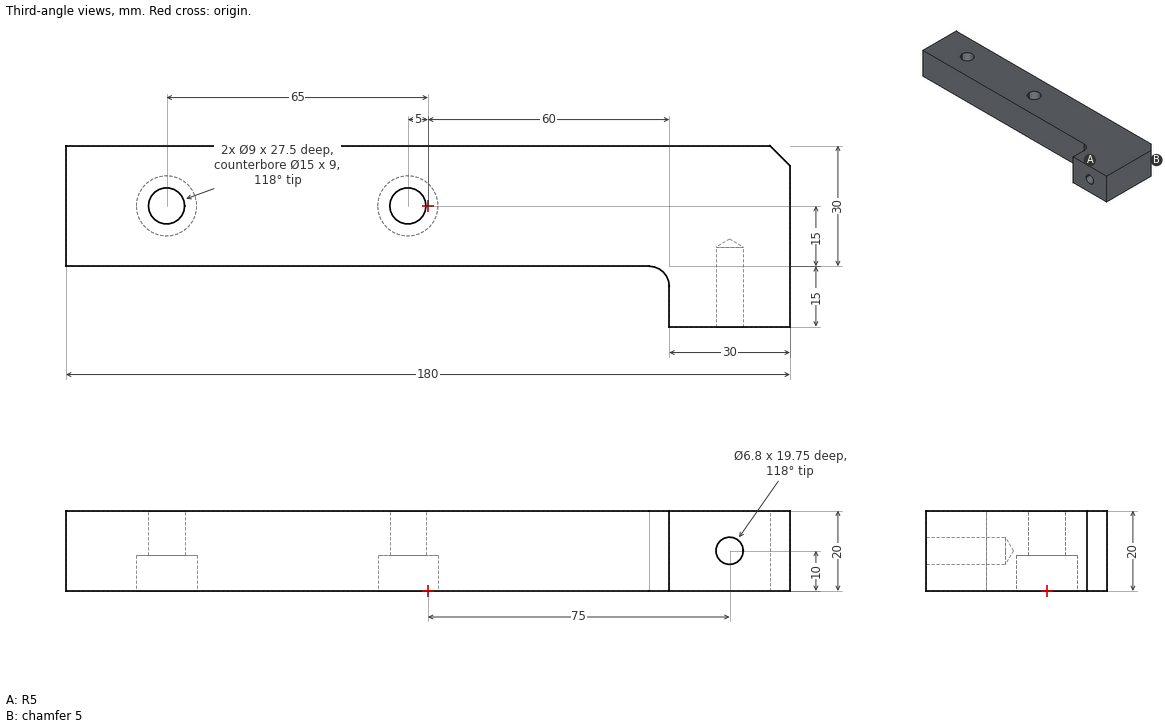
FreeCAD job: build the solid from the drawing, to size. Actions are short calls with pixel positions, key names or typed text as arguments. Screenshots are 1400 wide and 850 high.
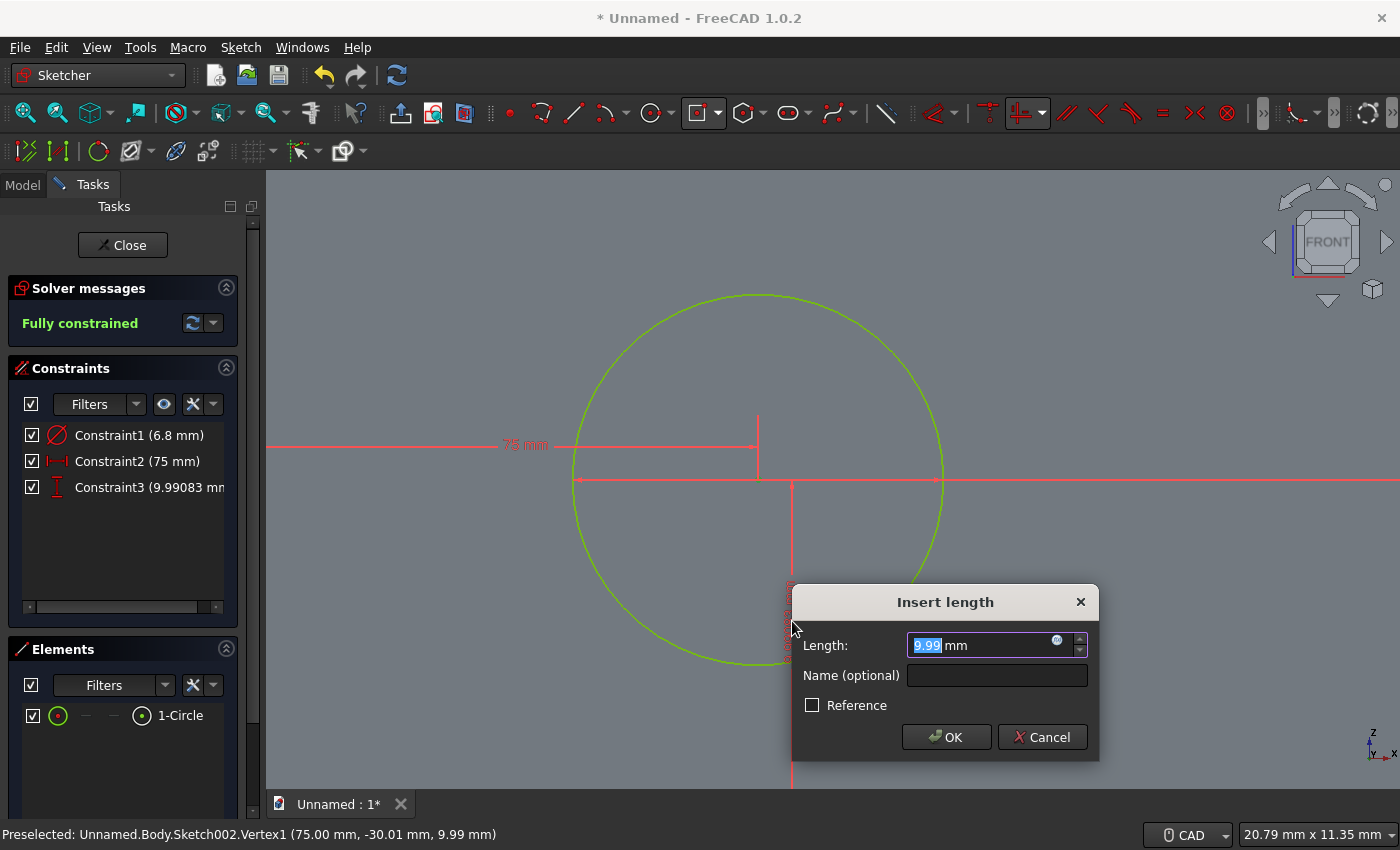
text(10)
key(Return)
key(Escape)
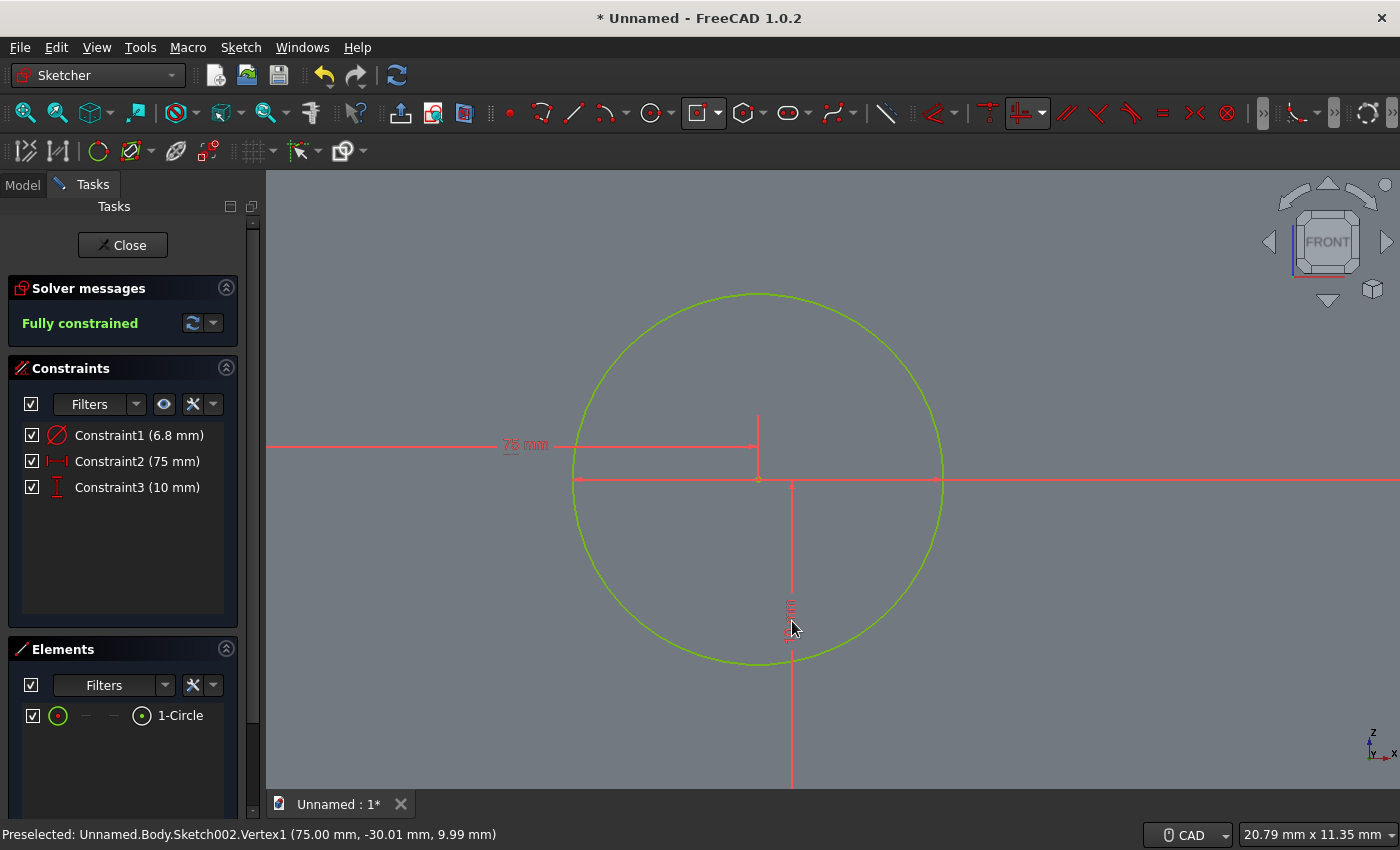
click(123, 245)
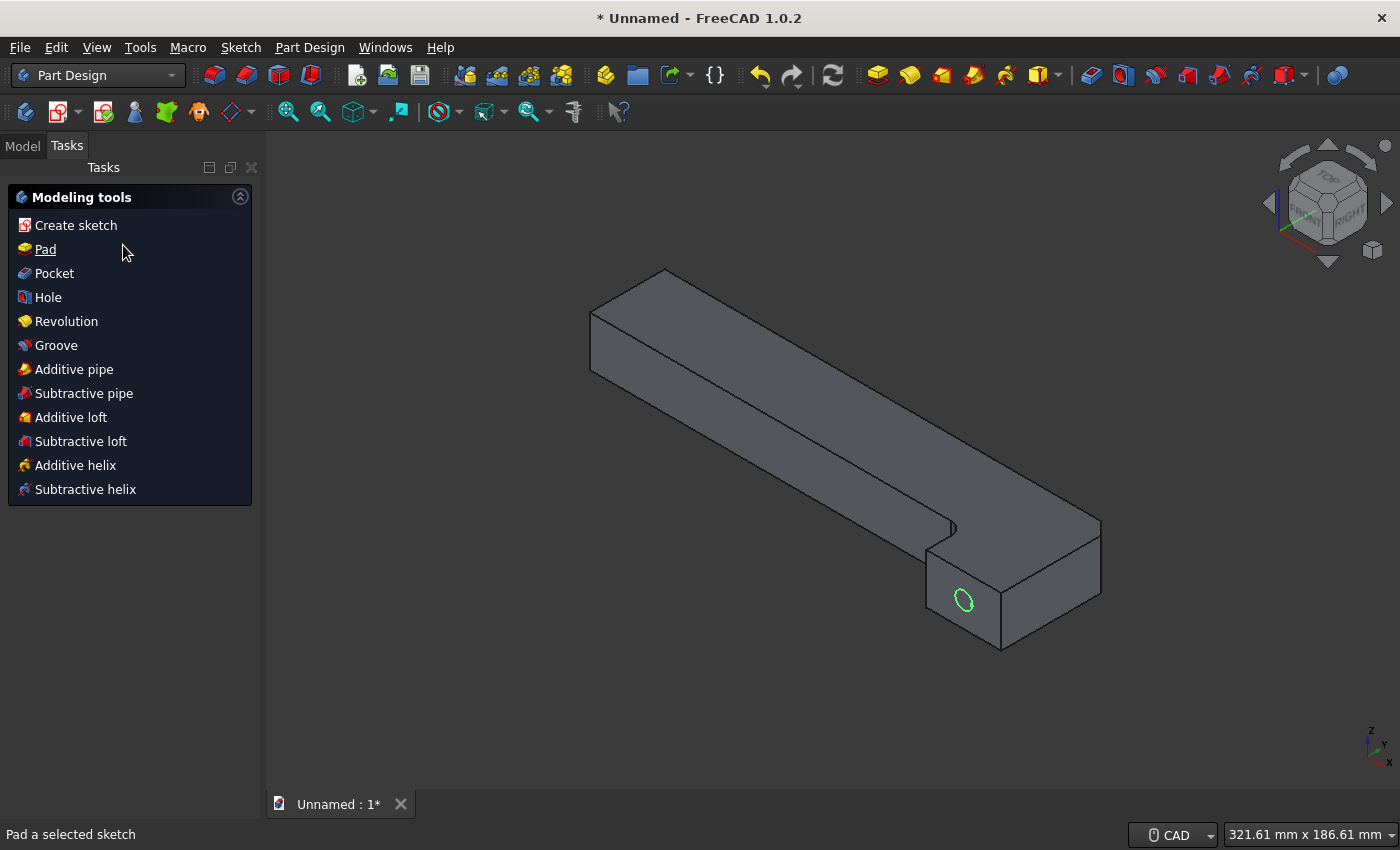
click(1124, 76)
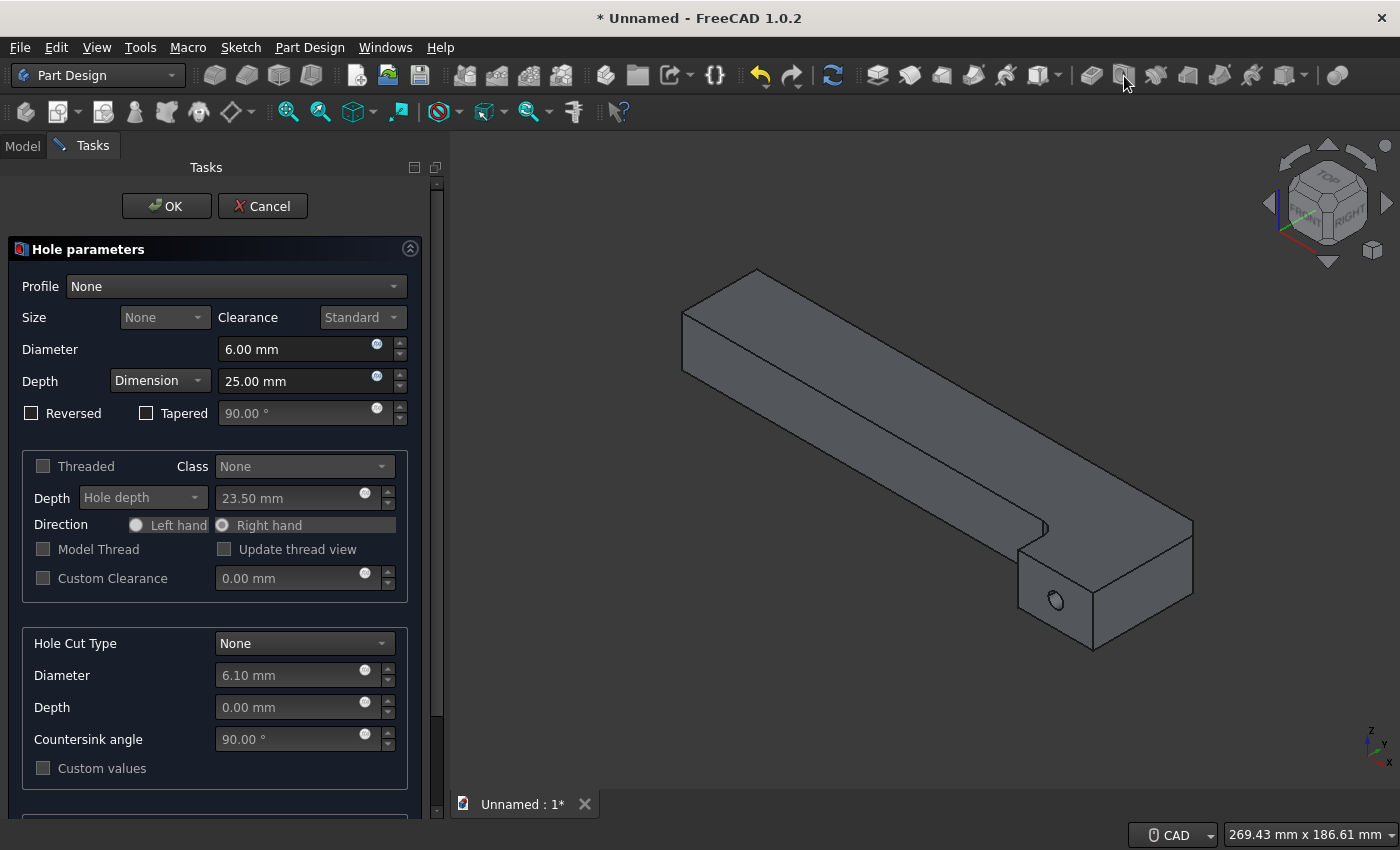
triple_click(305, 349)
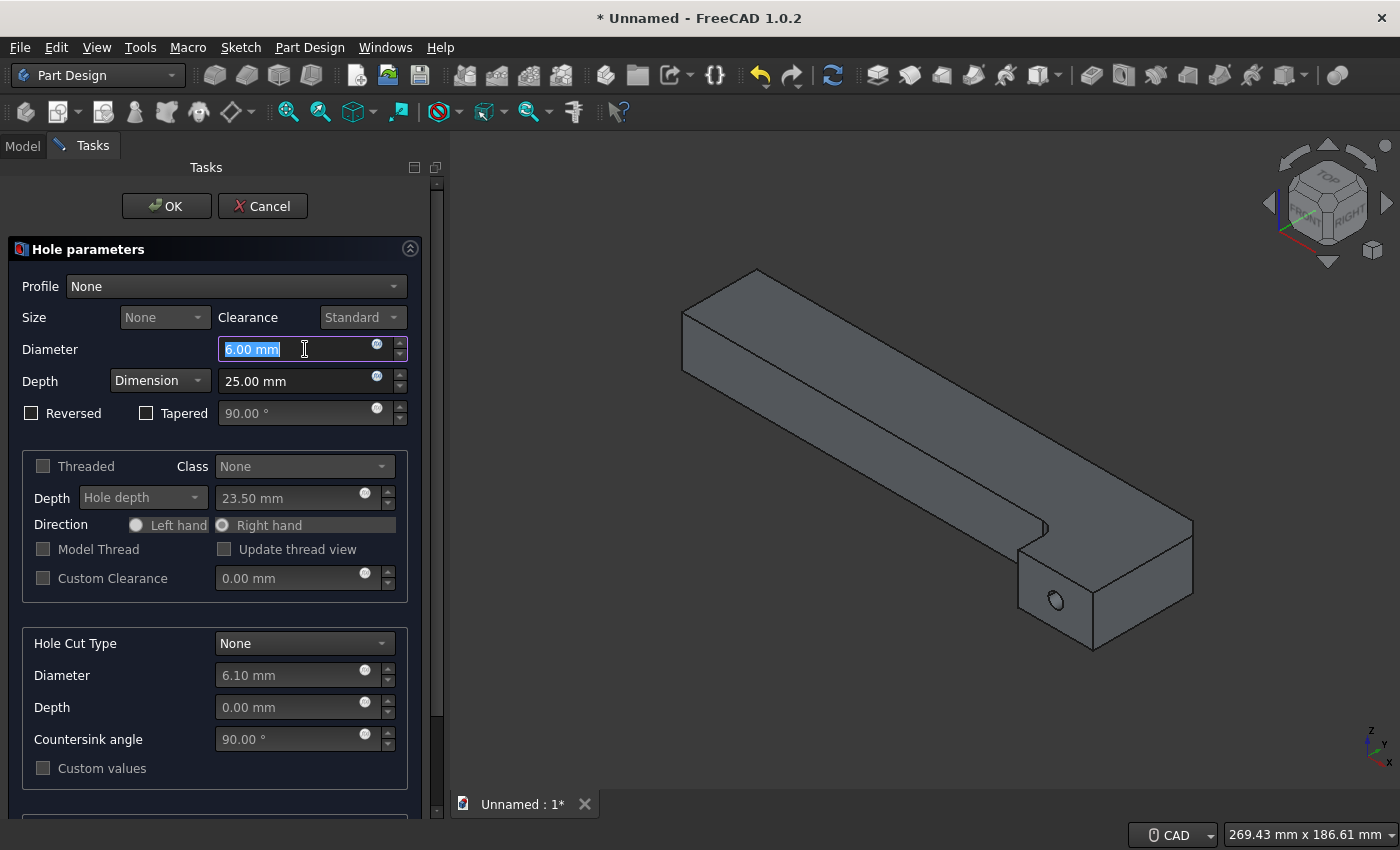
text(6.8)
key(Tab)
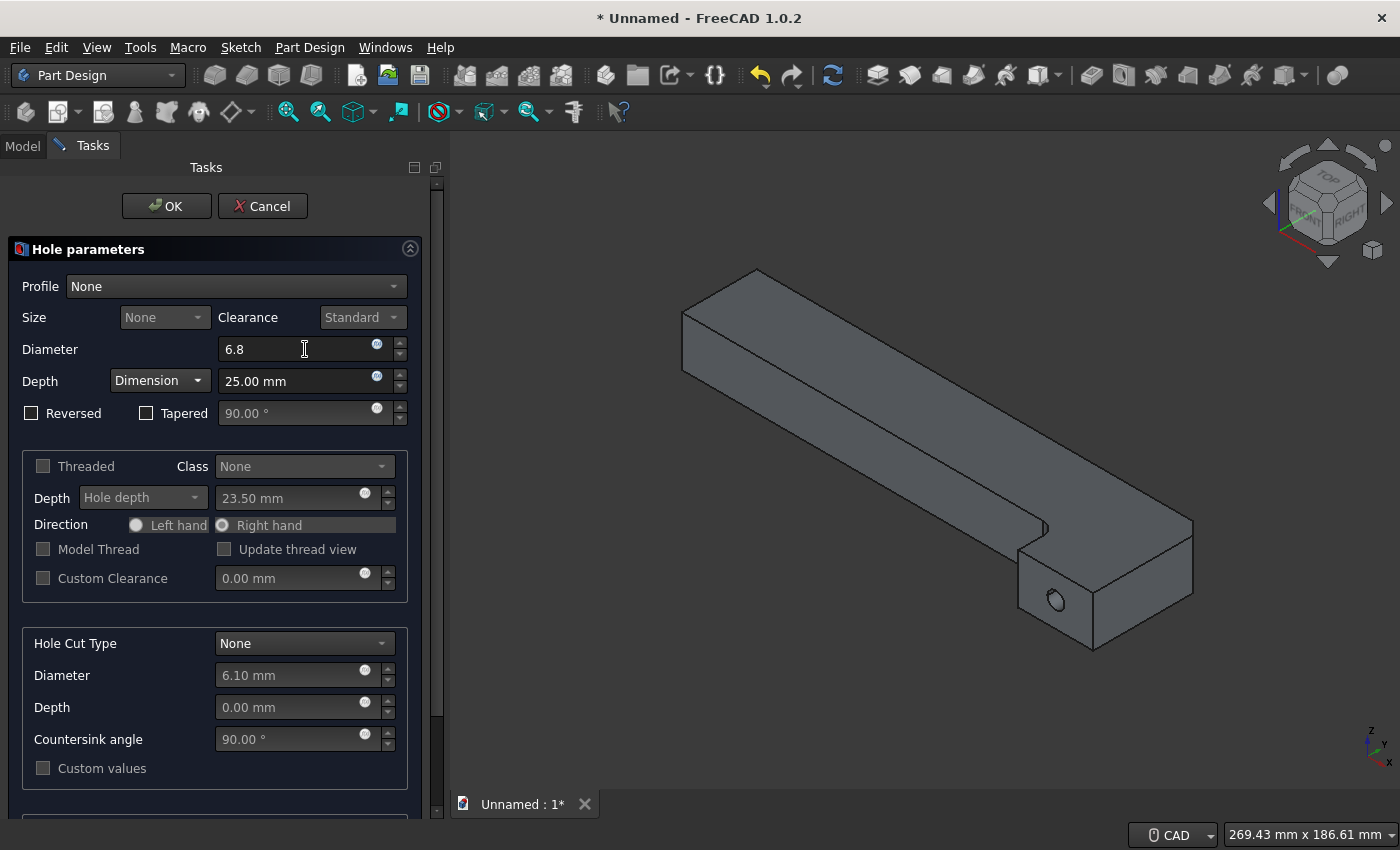
triple_click(305, 381)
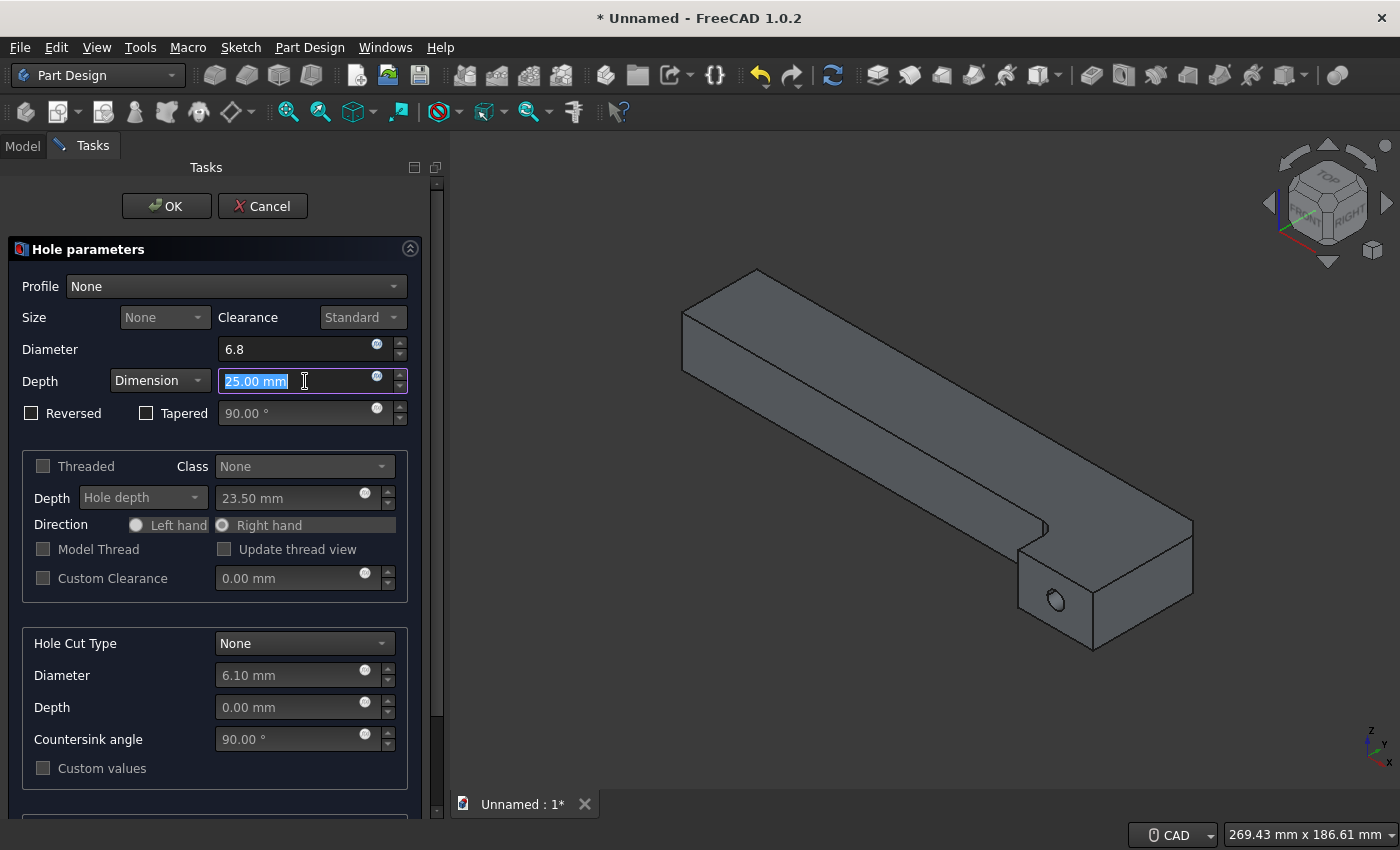
text(19.75)
key(Tab)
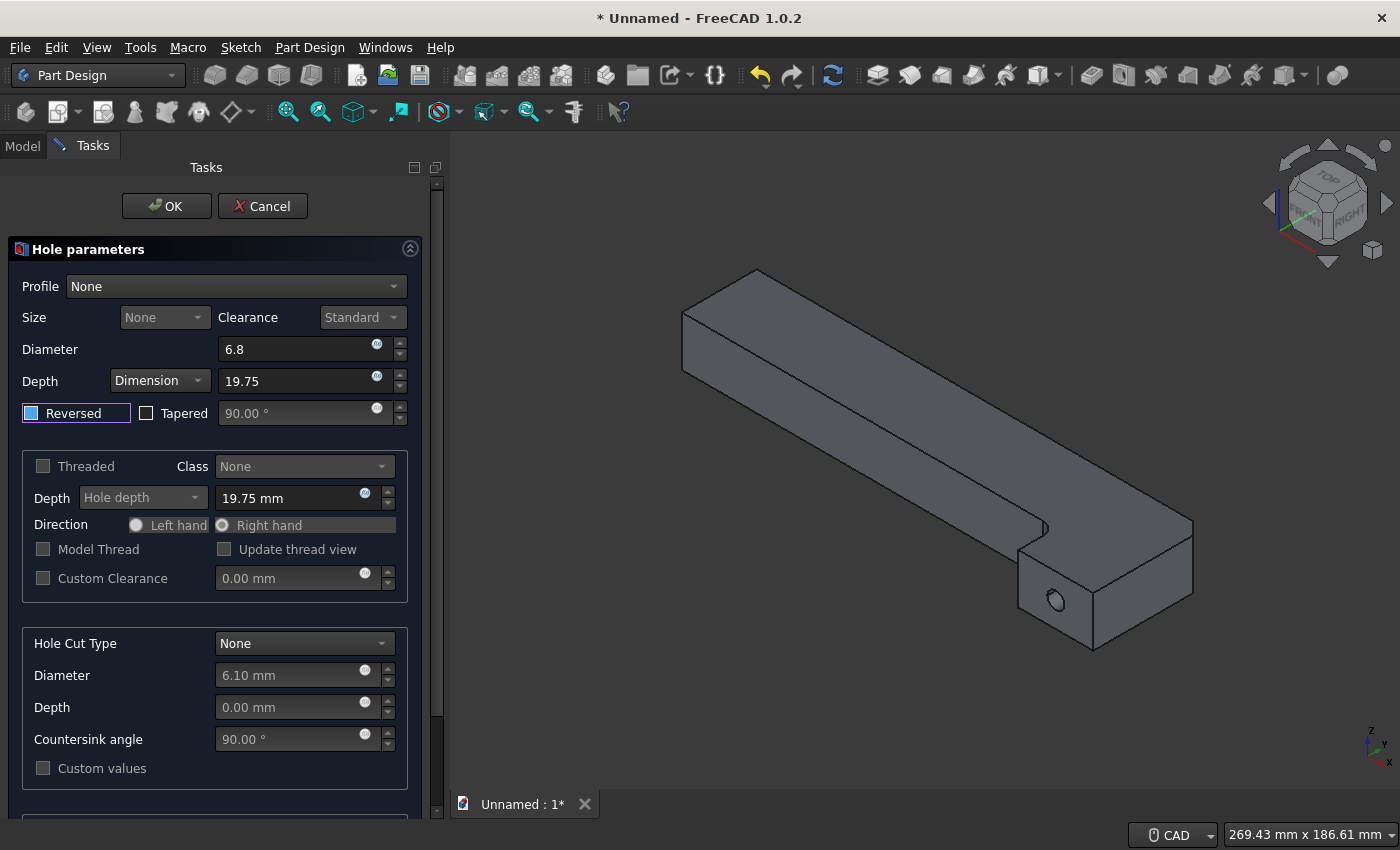
click(167, 206)